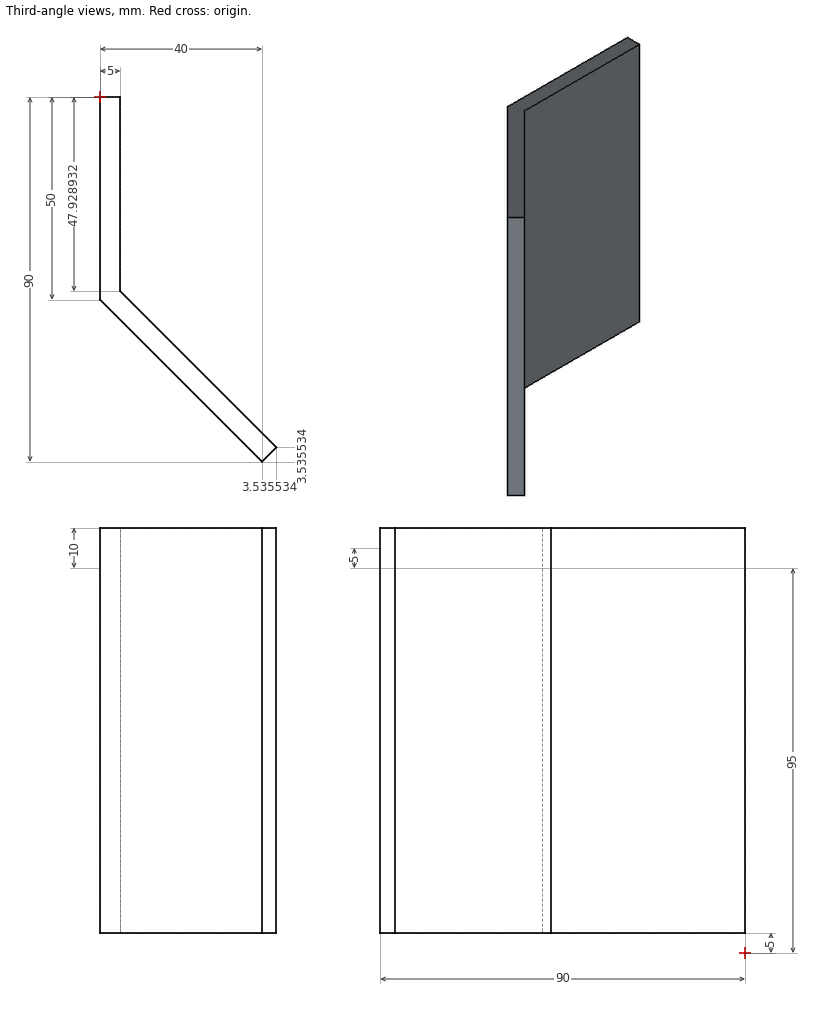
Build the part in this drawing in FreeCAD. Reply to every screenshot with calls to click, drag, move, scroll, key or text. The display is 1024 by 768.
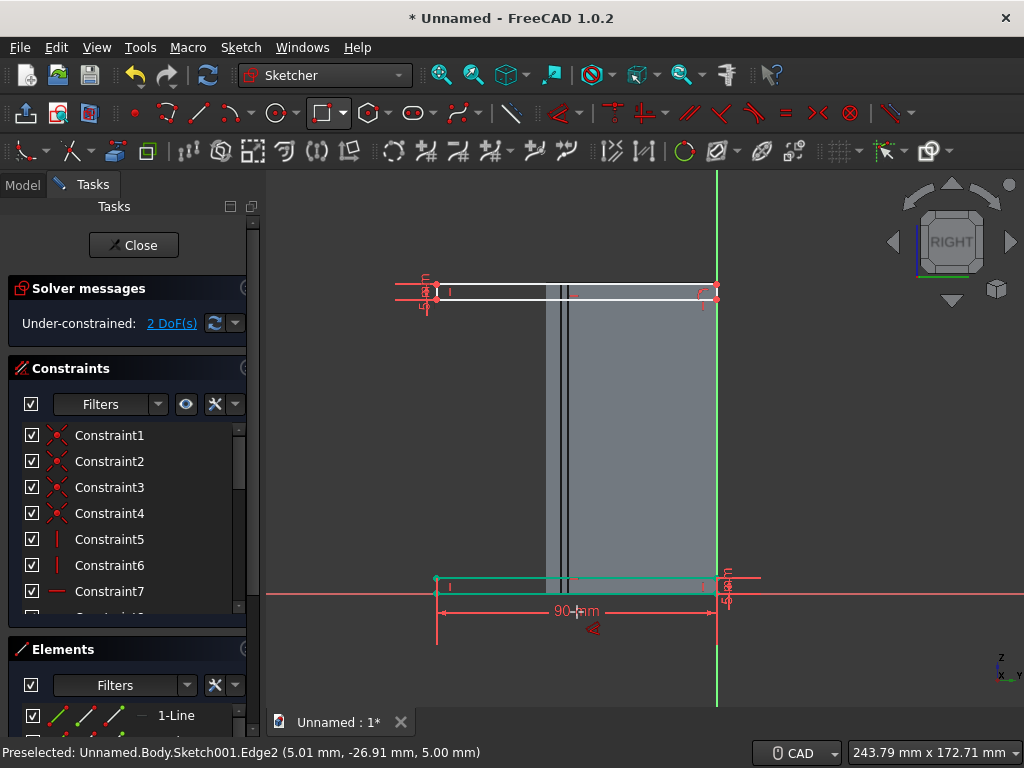
click(521, 300)
click(577, 266)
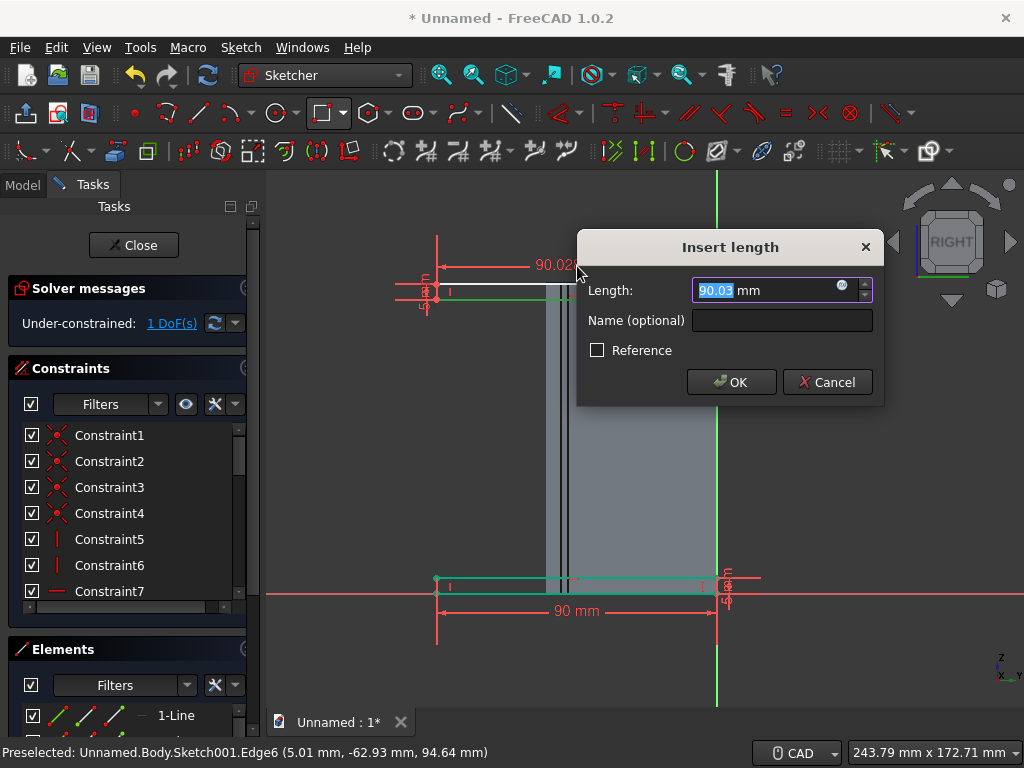
text(90)
key(Return)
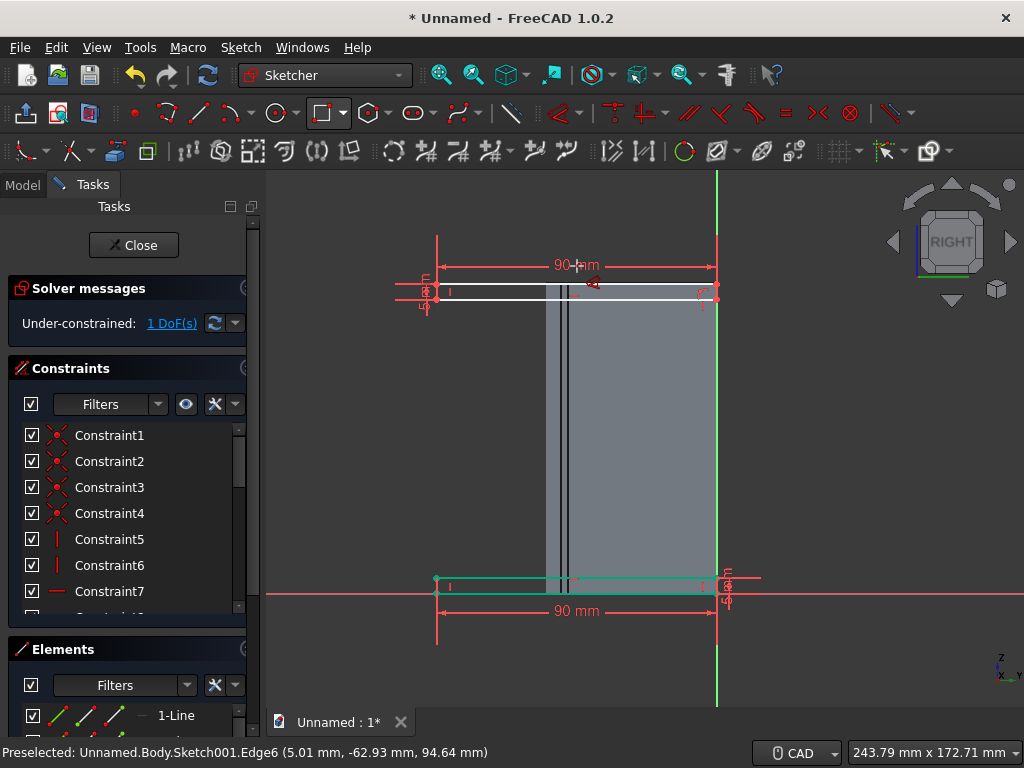
click(437, 300)
click(751, 447)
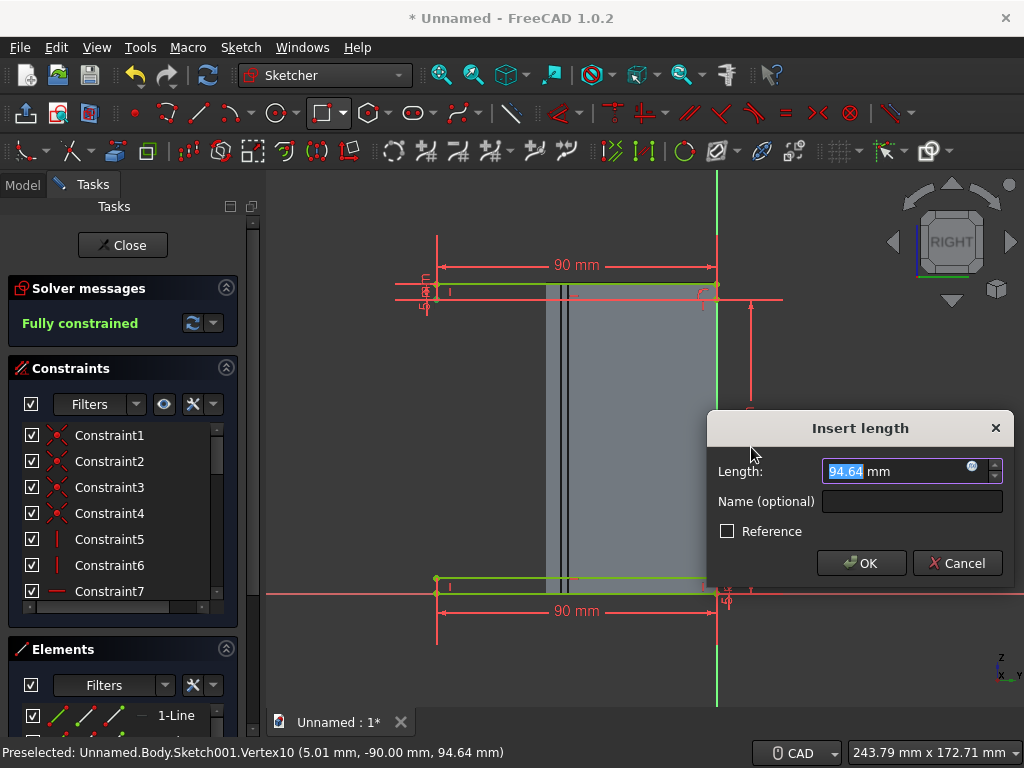
text(95)
key(Return)
key(Escape)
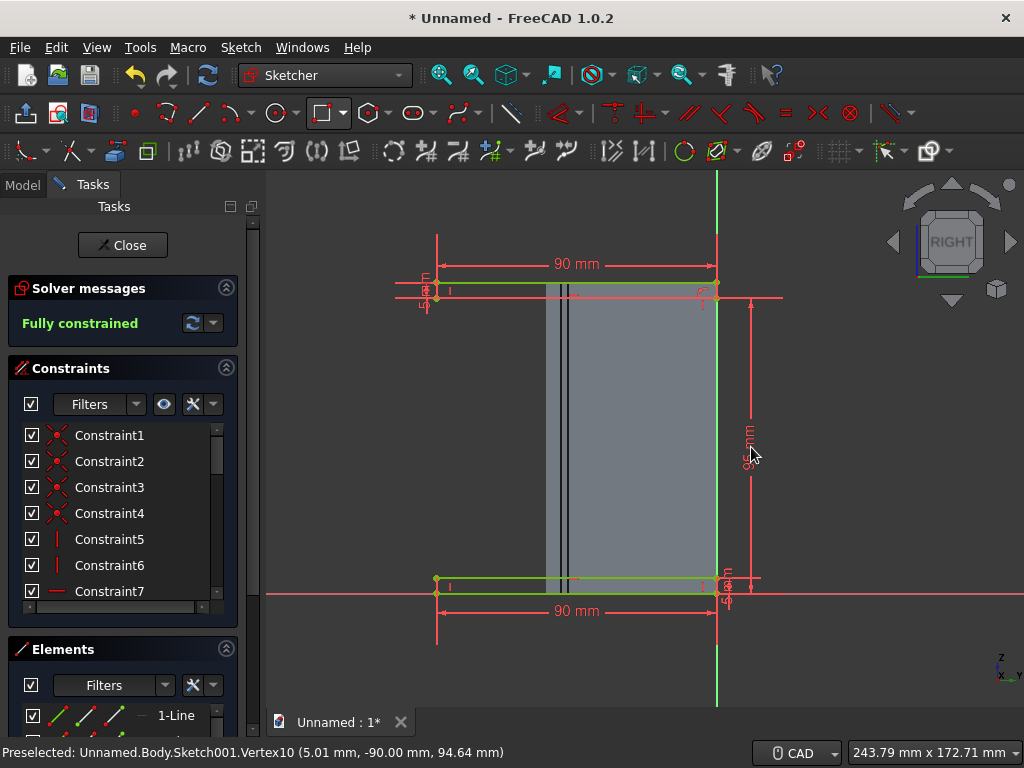
click(123, 245)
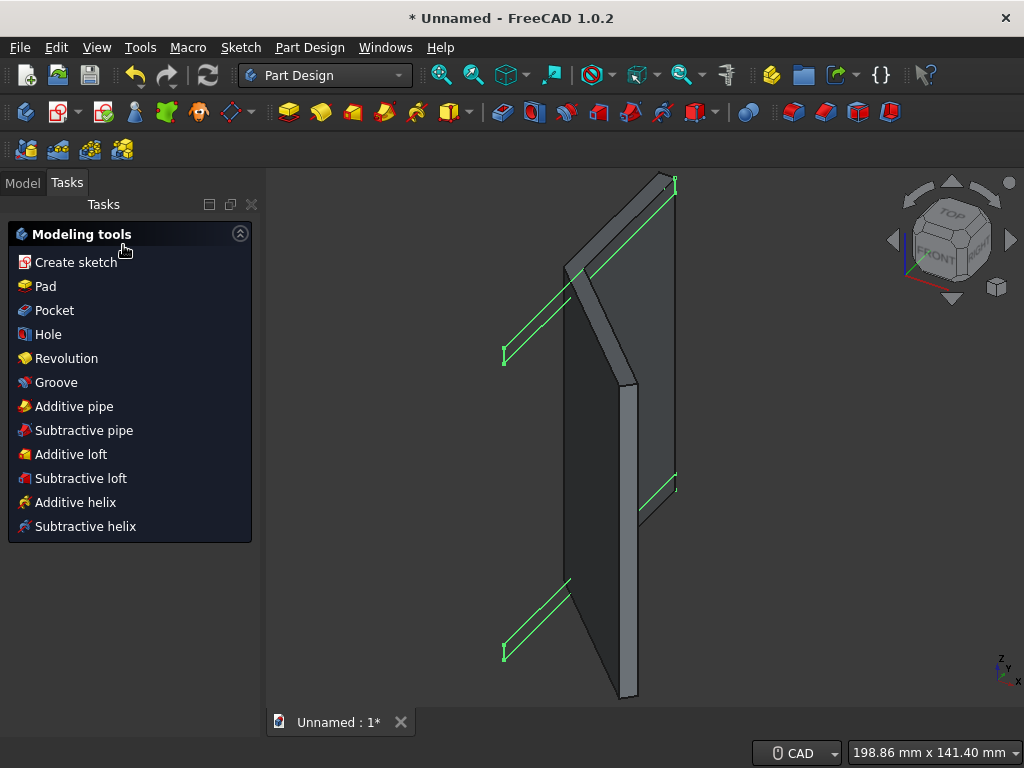
click(504, 112)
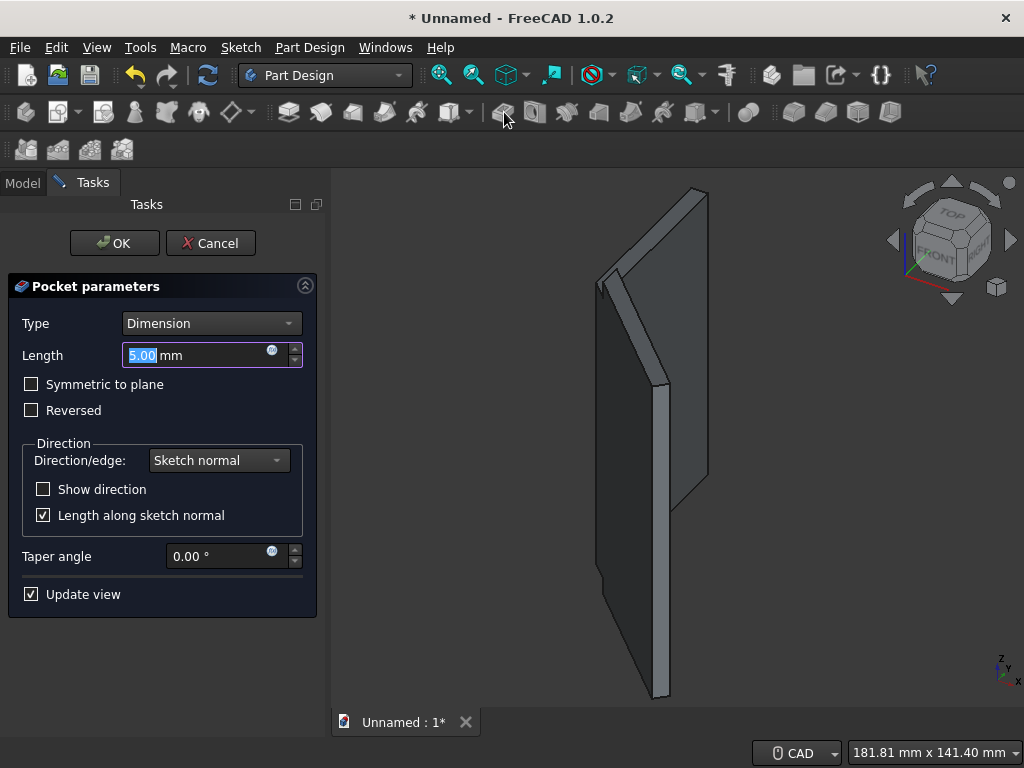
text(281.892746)
key(Tab)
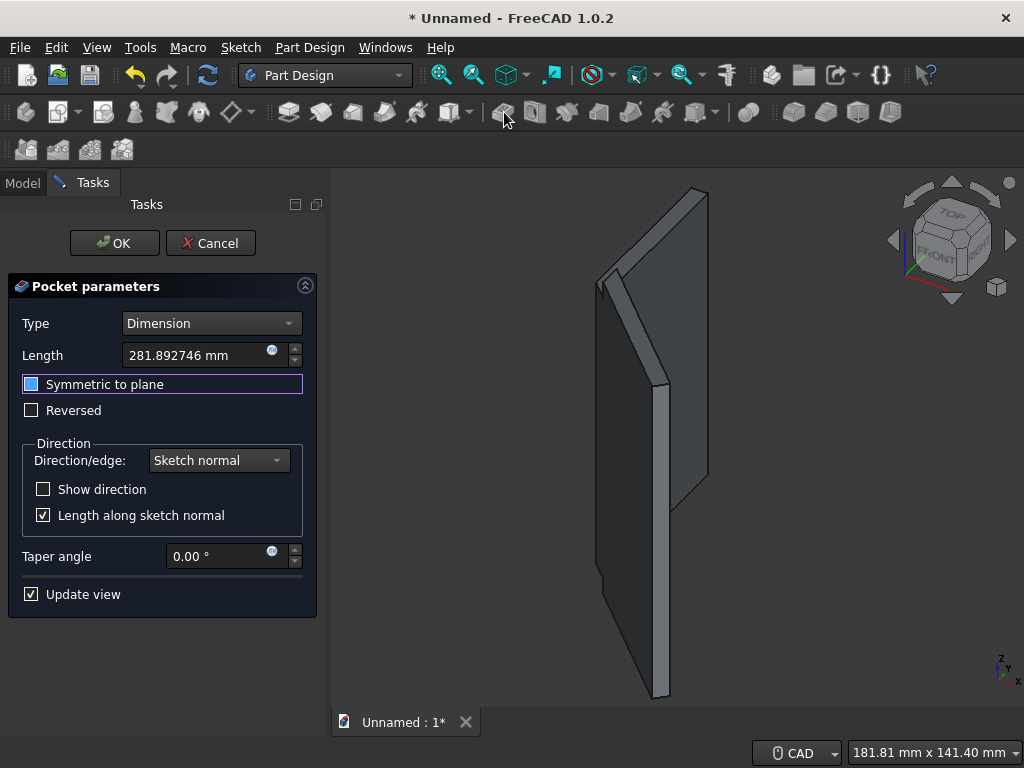
click(30, 384)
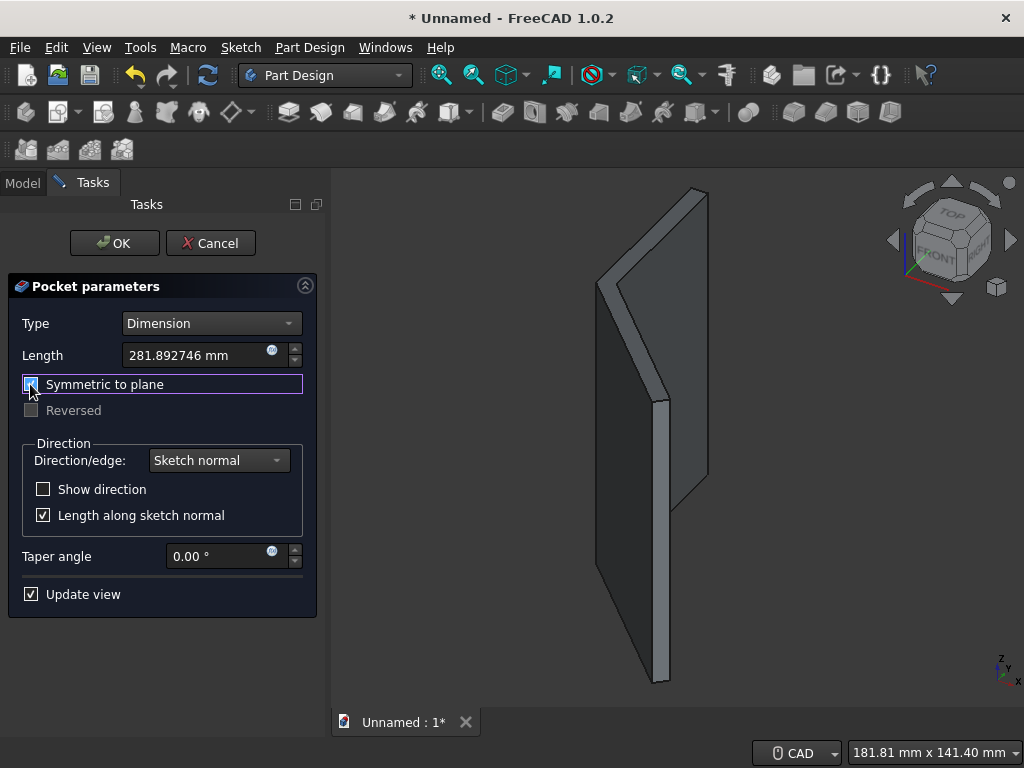
click(115, 243)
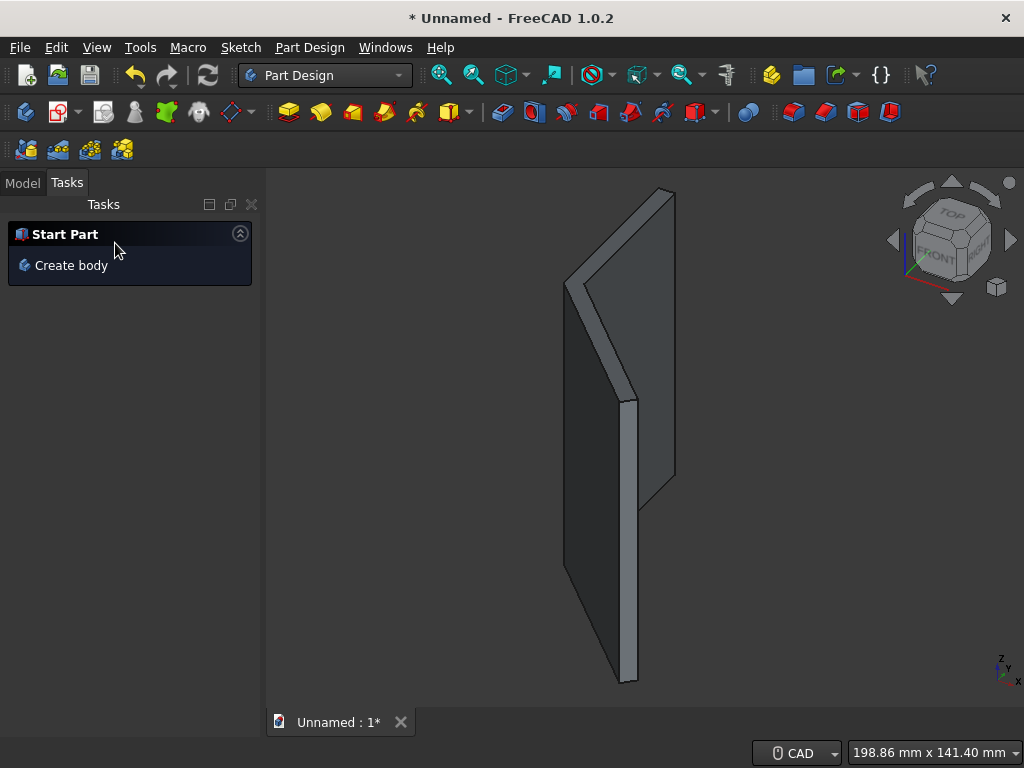
key(0)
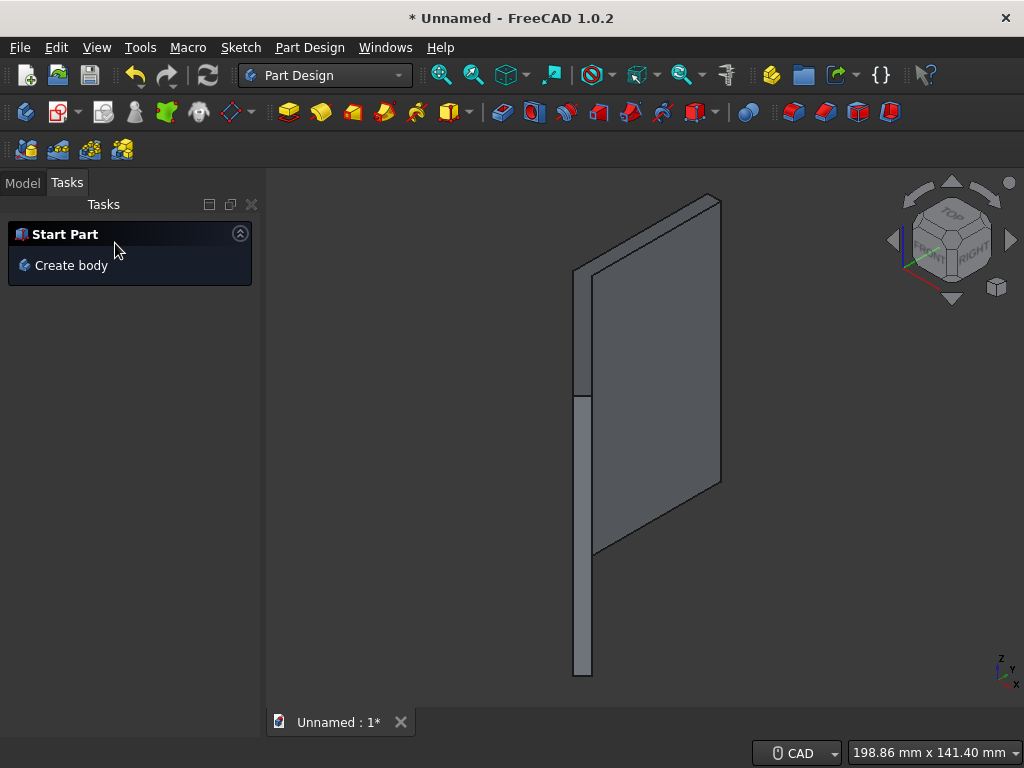
key(2)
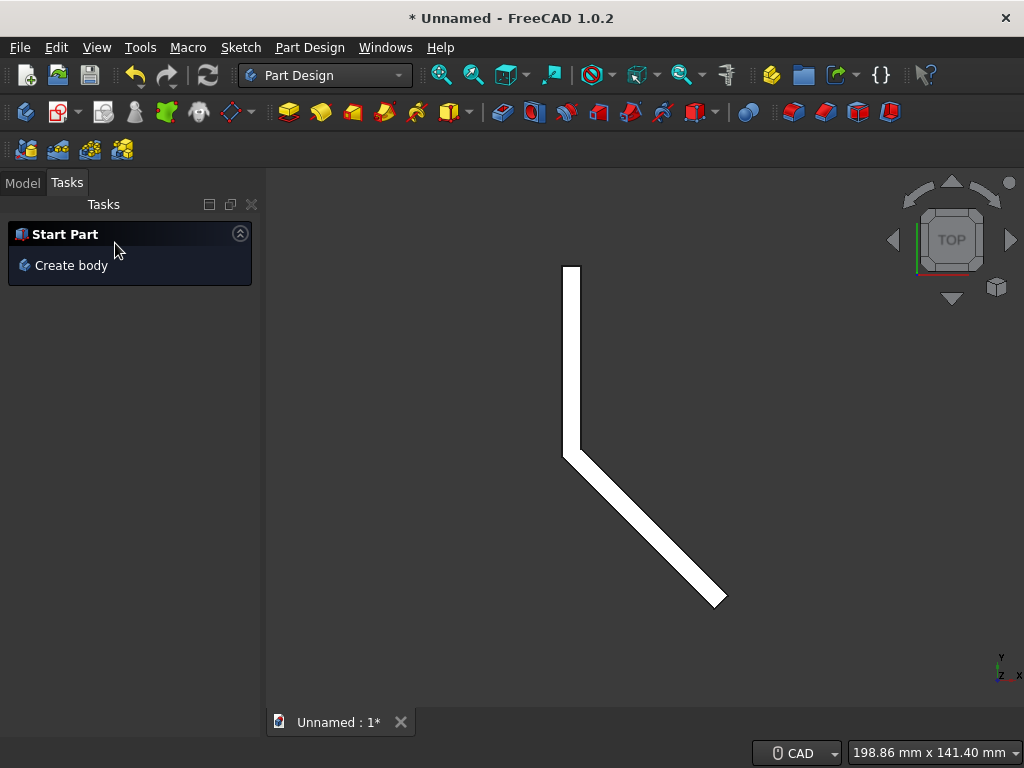
key(1)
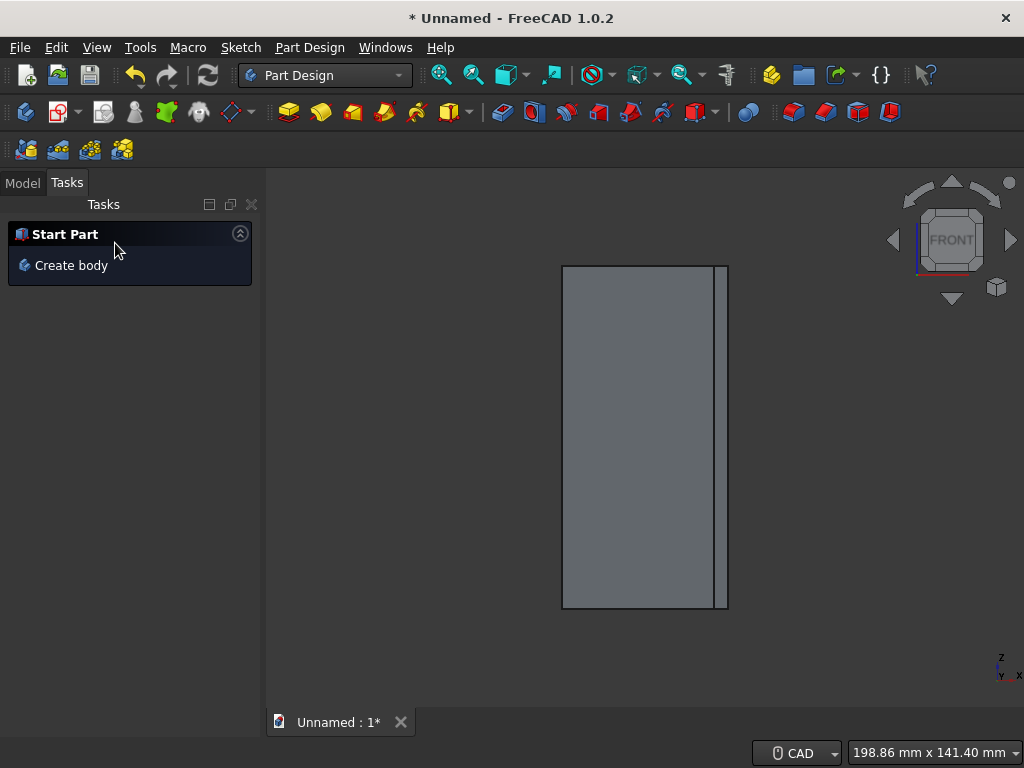
click(23, 182)